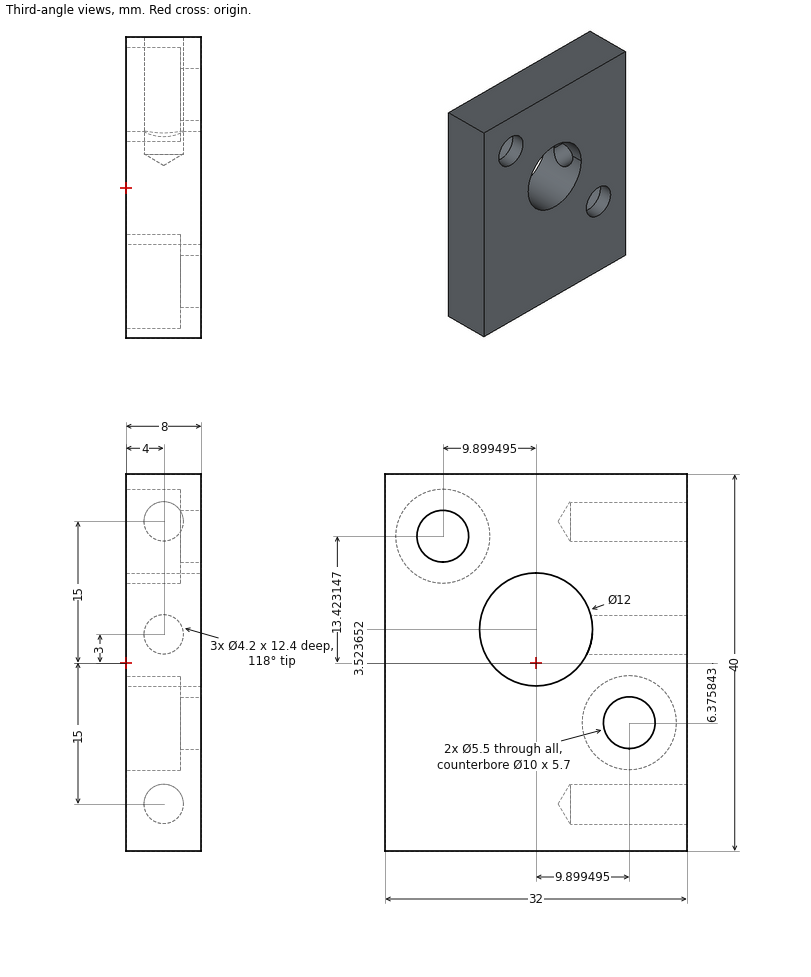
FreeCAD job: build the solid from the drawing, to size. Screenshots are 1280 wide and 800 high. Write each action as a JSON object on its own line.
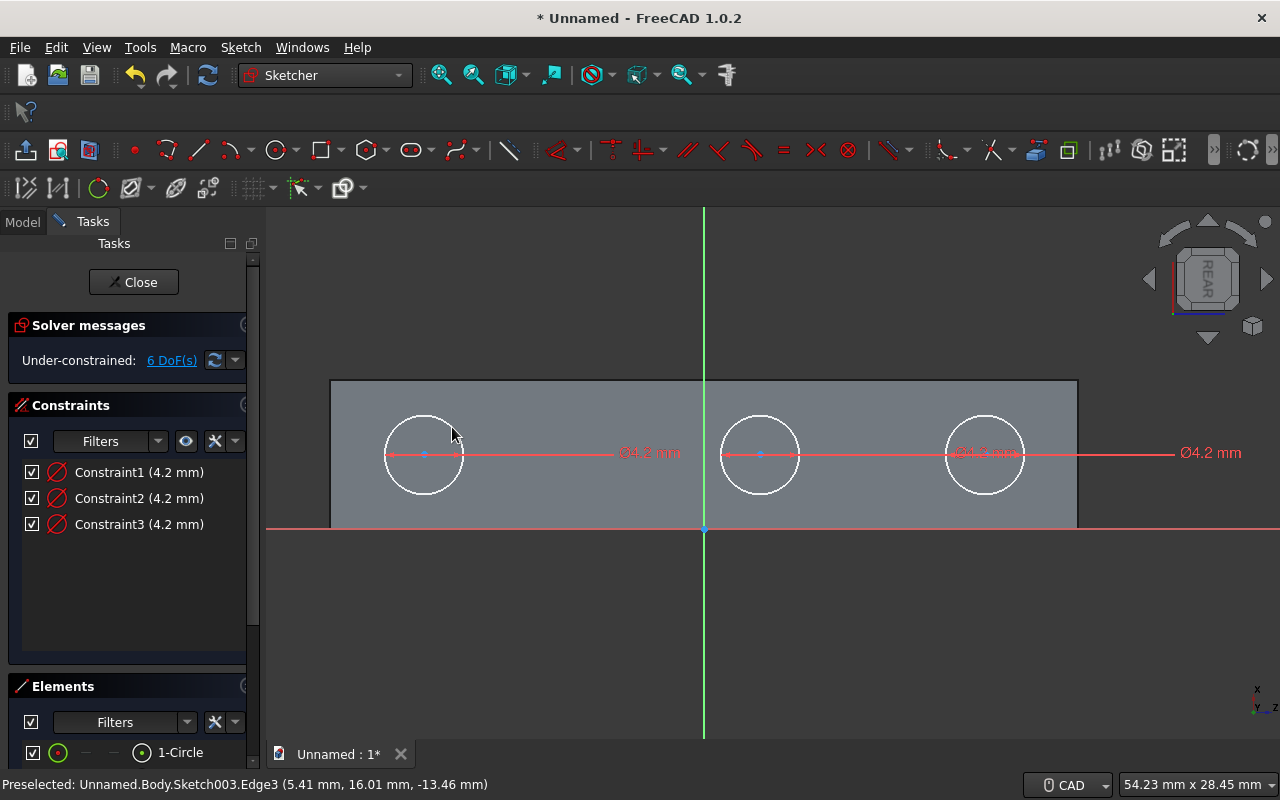
{"action": "left_click", "coordinate": [760, 455]}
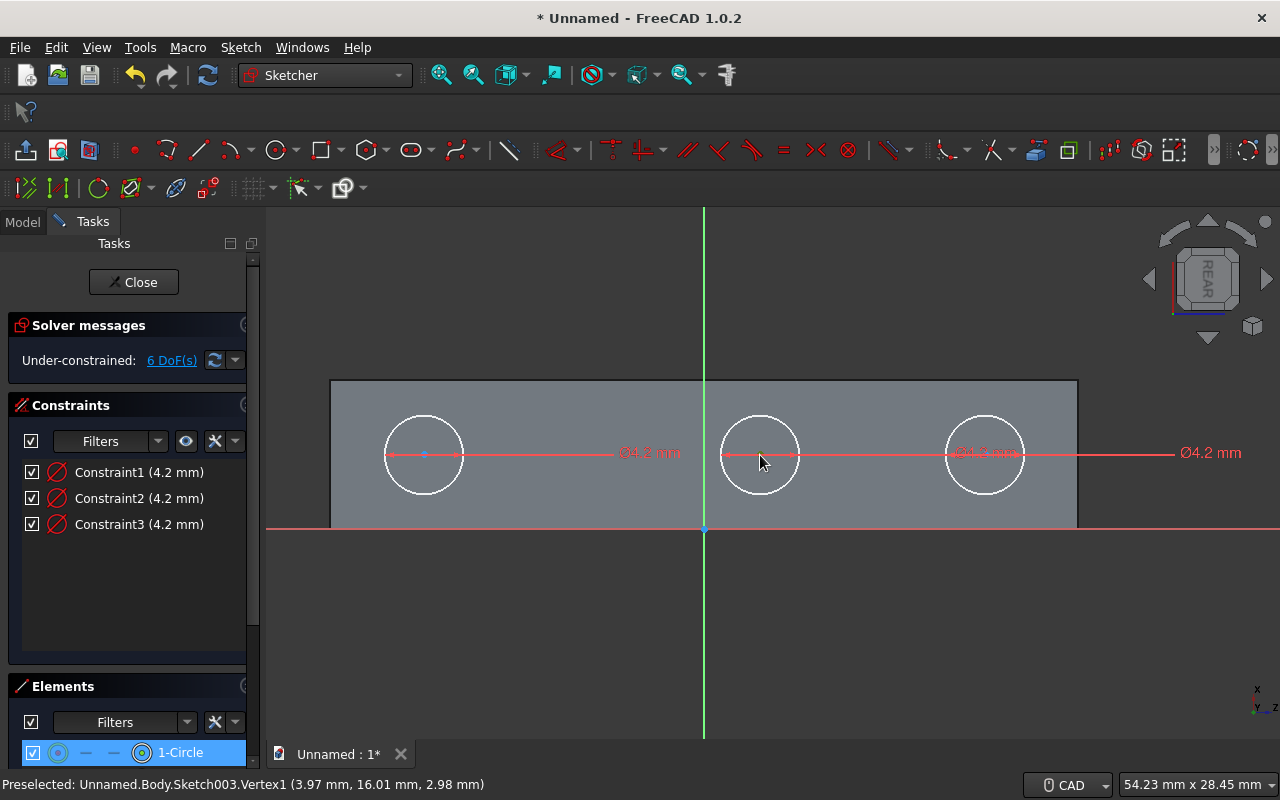
{"action": "left_click", "coordinate": [985, 455]}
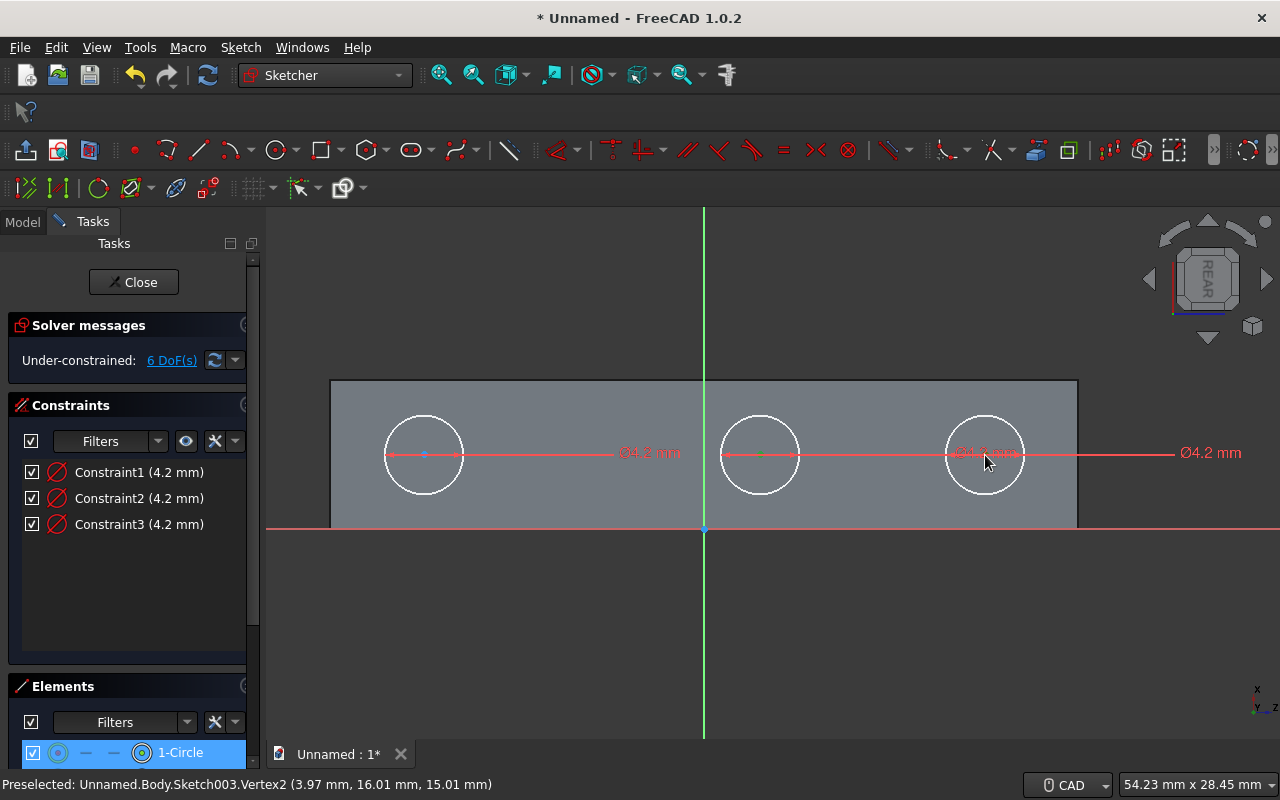
{"action": "key", "text": "h"}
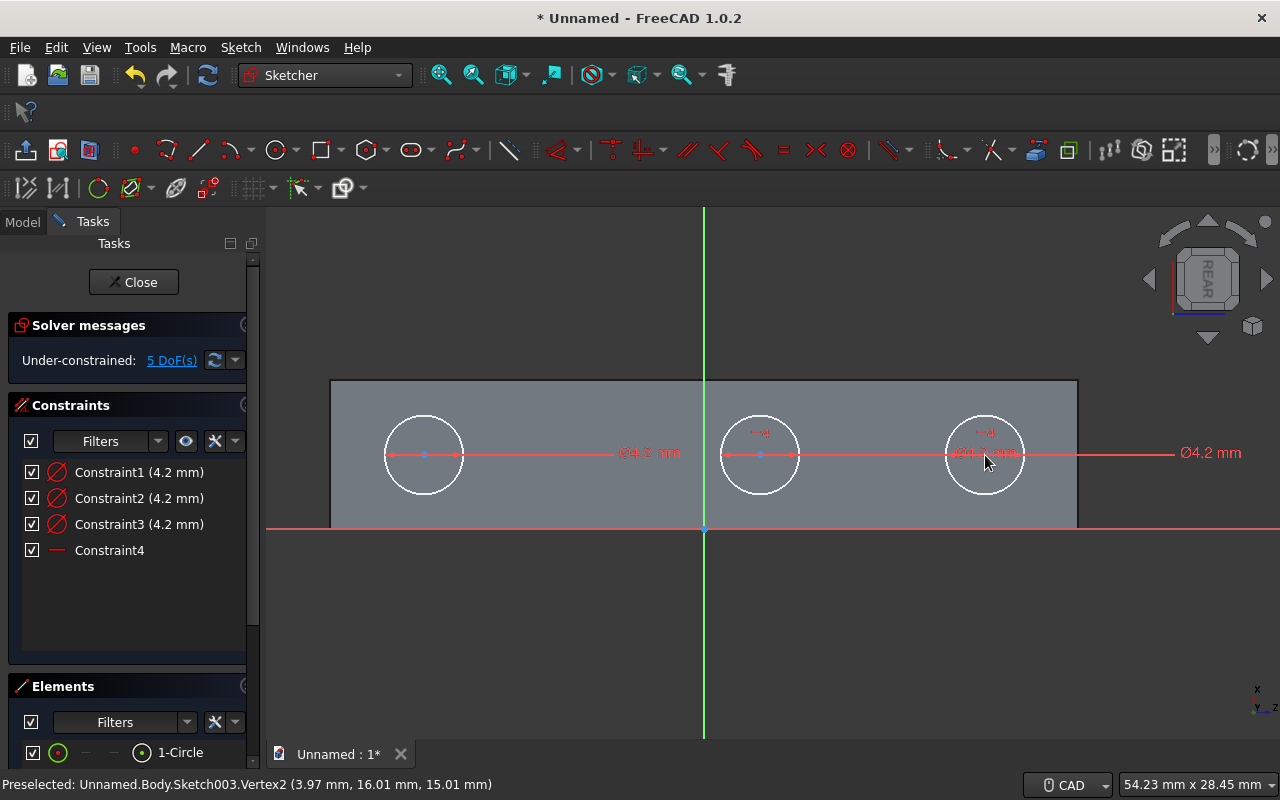
{"action": "left_click", "coordinate": [760, 455]}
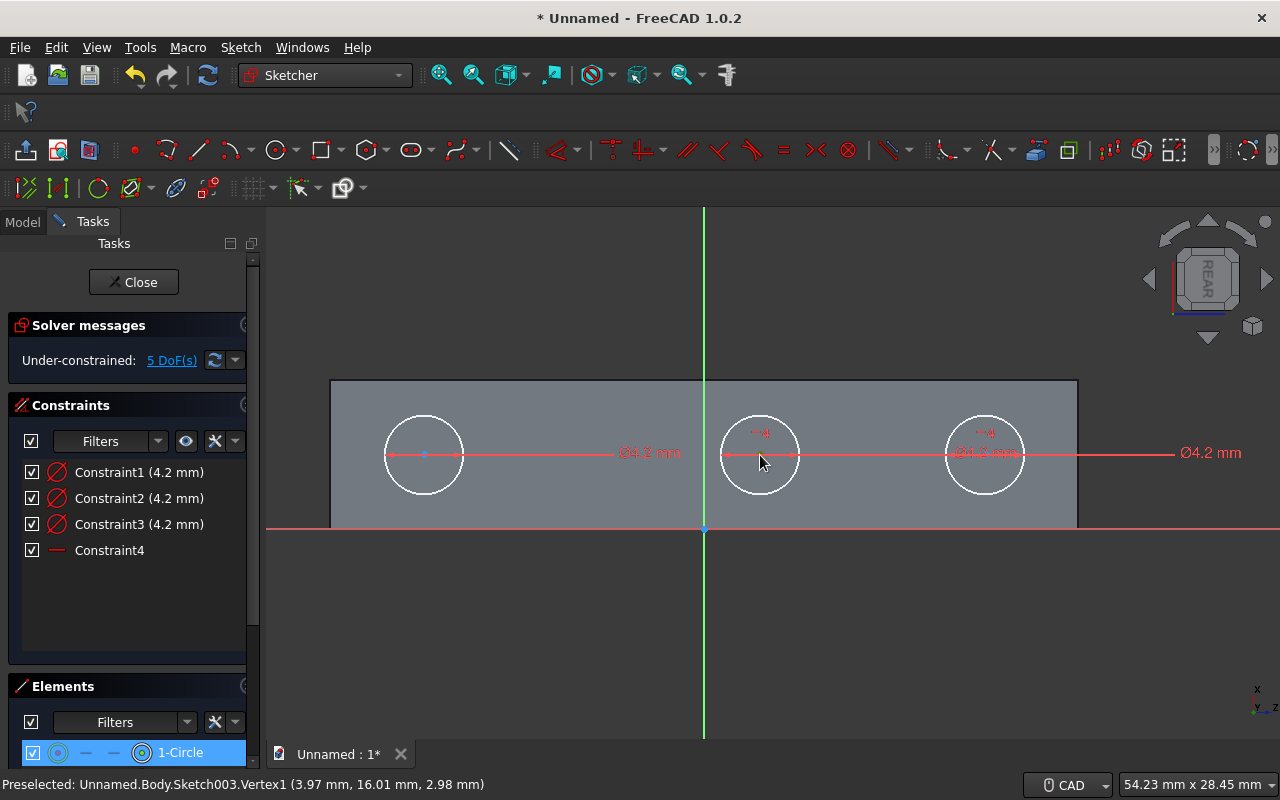
{"action": "left_click", "coordinate": [424, 455]}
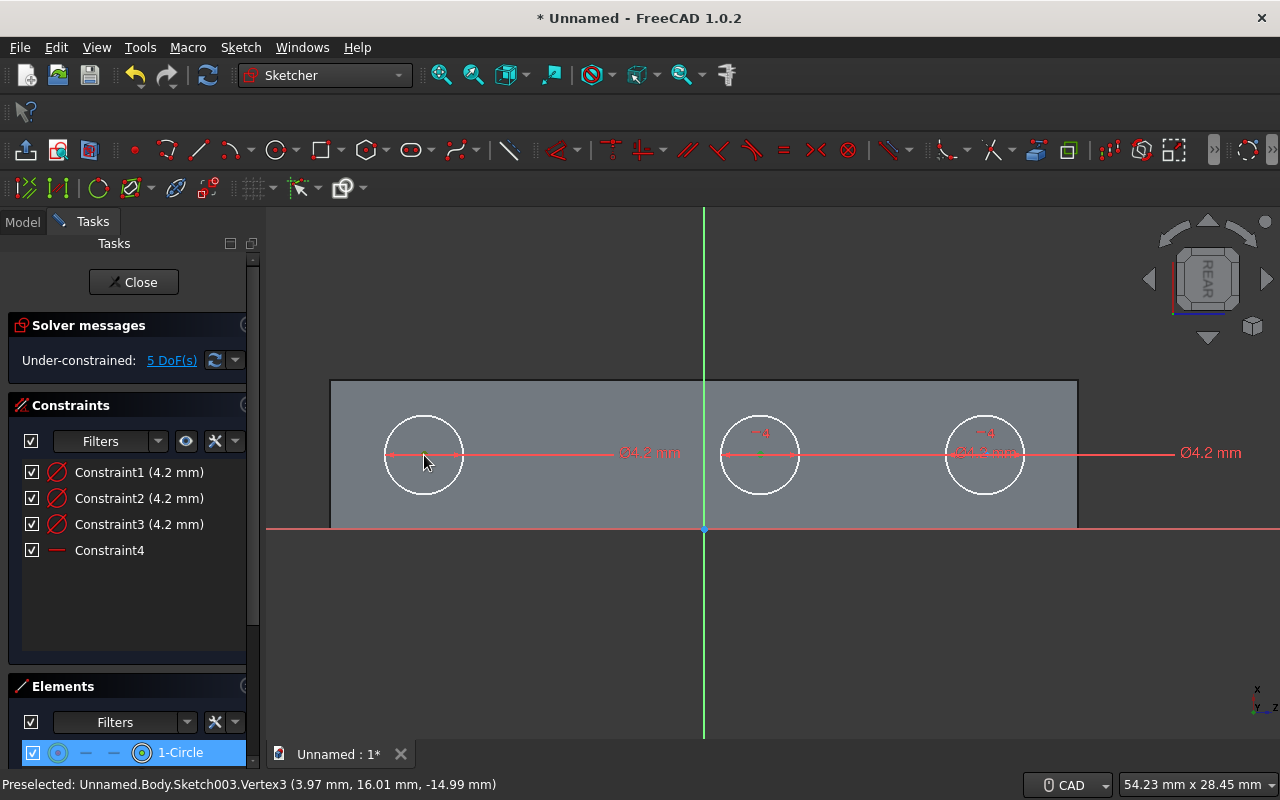
{"action": "key", "text": "h"}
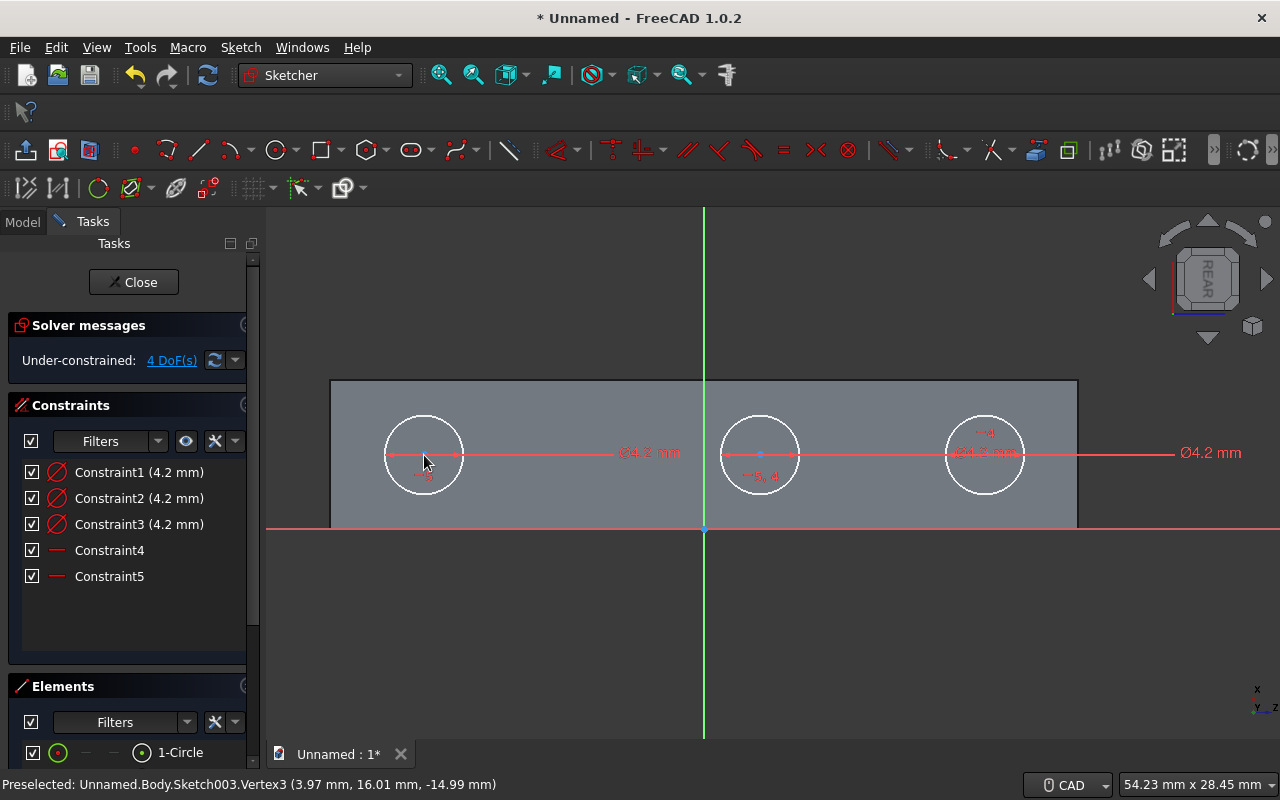
{"action": "key", "text": "d"}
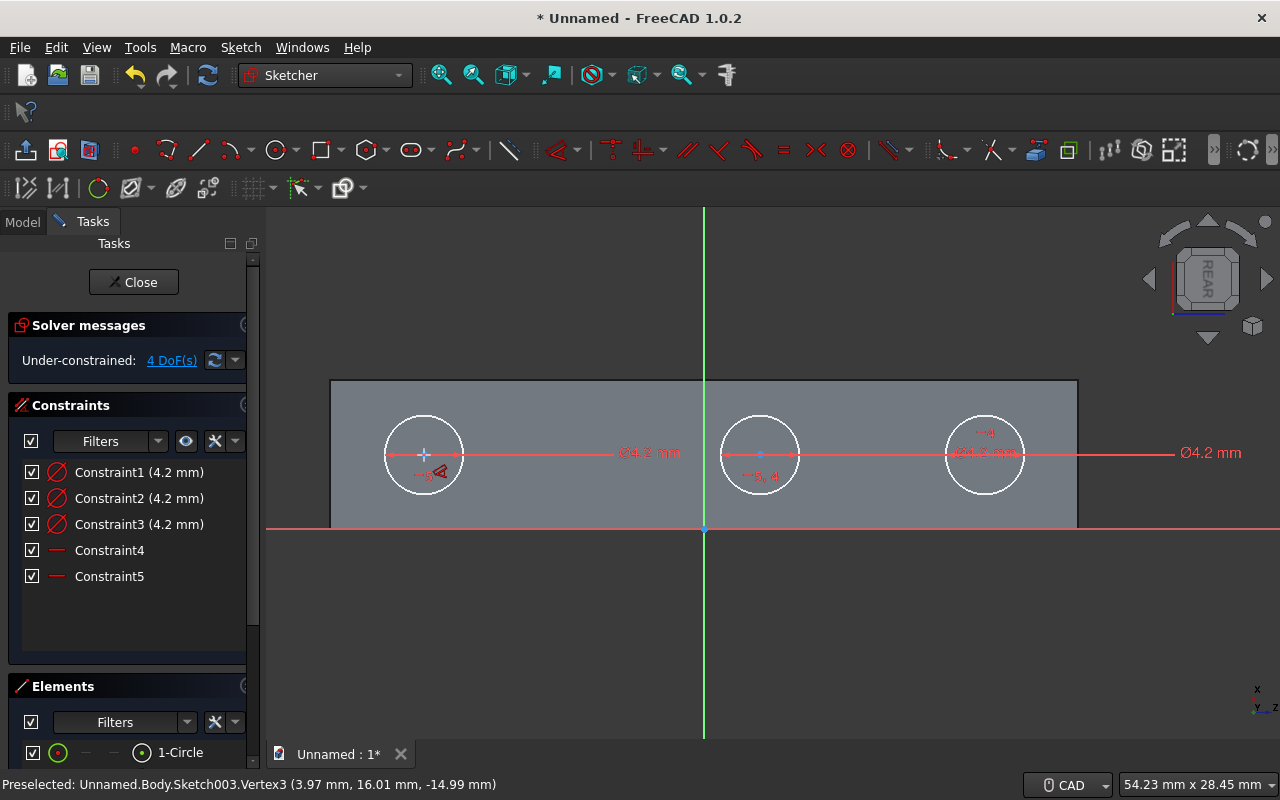
{"action": "left_click", "coordinate": [760, 455]}
{"action": "left_click", "coordinate": [732, 563]}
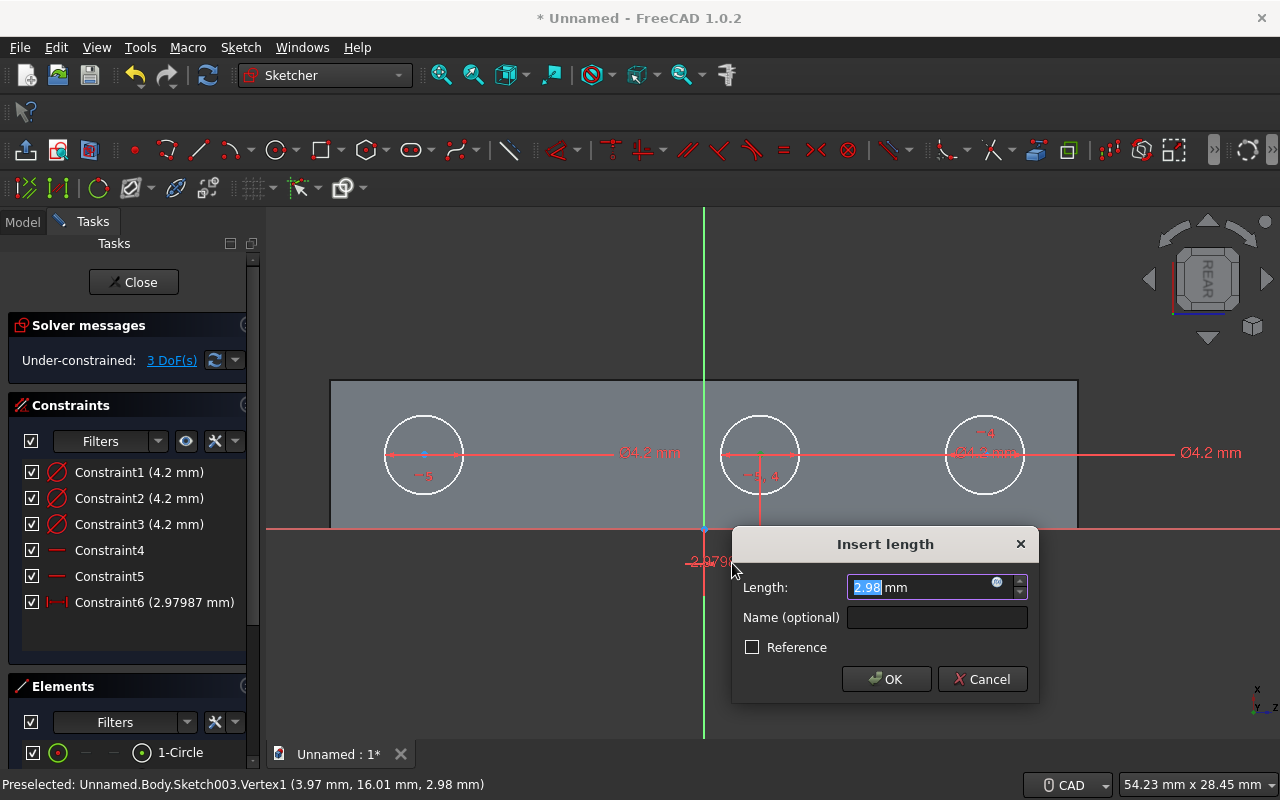
{"action": "type", "text": "3"}
{"action": "key", "text": "Return"}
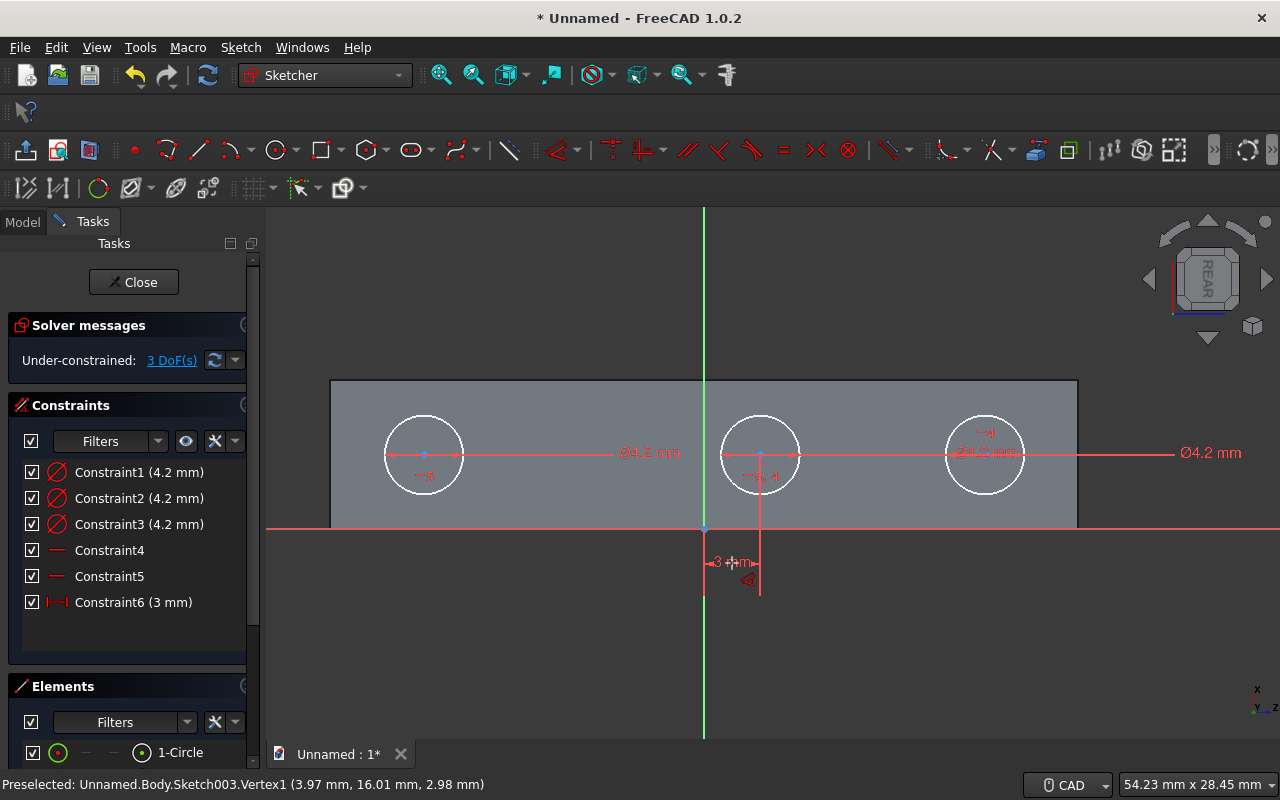
{"action": "left_click", "coordinate": [760, 455]}
{"action": "left_click", "coordinate": [794, 509]}